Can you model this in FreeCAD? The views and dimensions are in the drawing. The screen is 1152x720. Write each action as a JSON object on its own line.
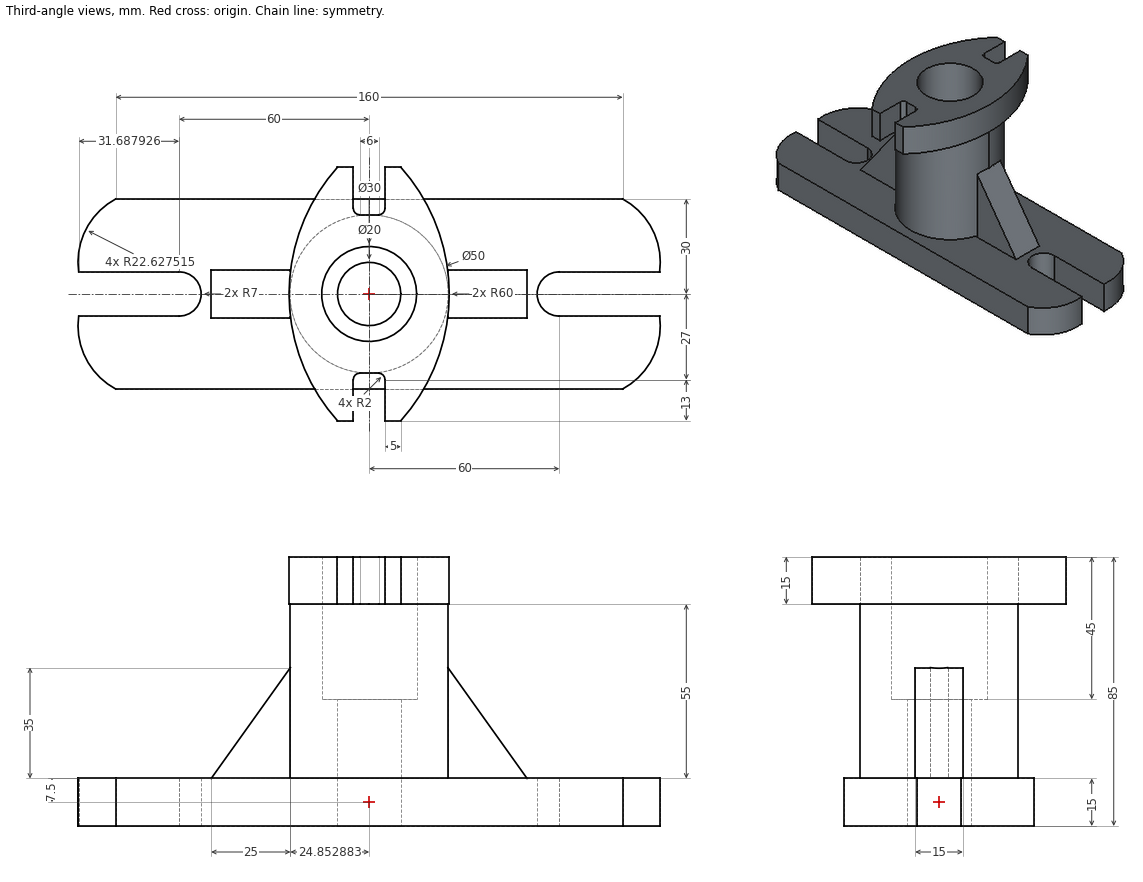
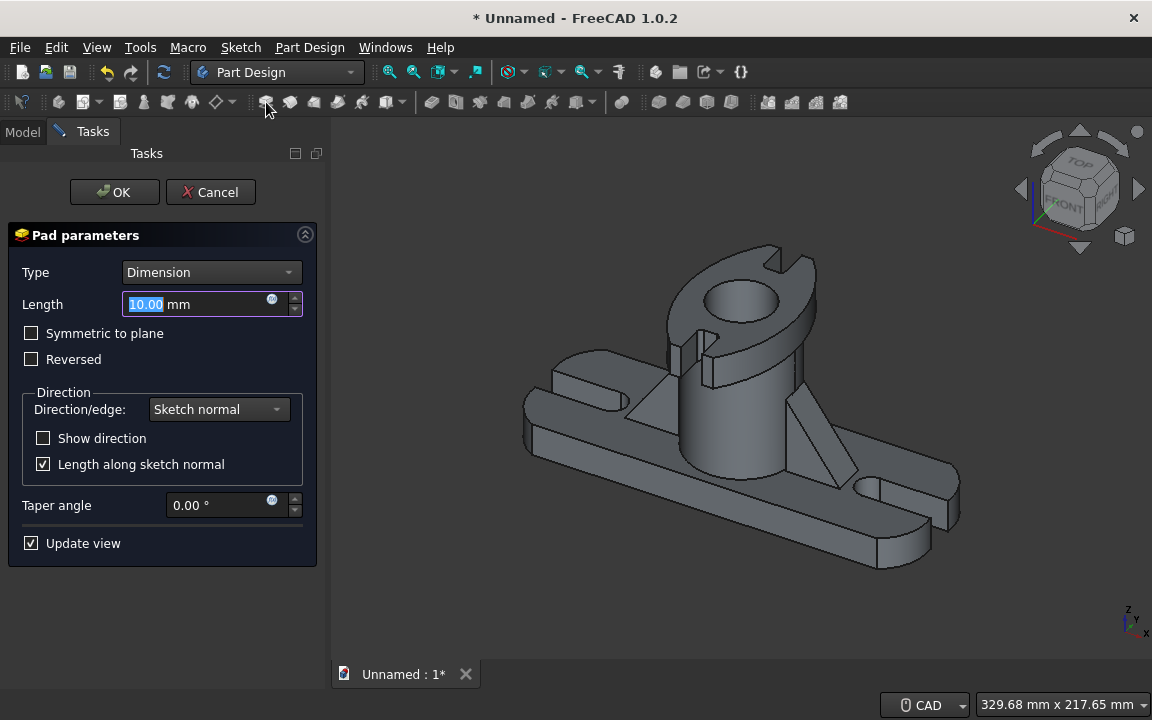
{"action": "type", "text": "85"}
{"action": "key", "text": "Tab"}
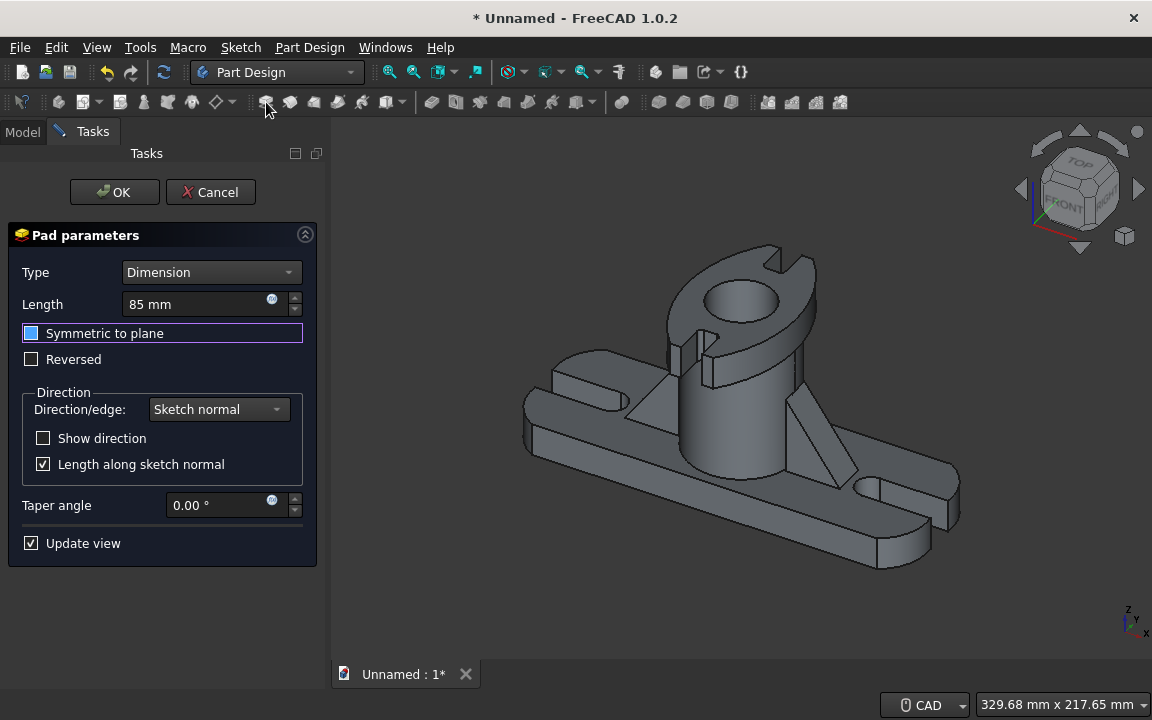
{"action": "left_click", "coordinate": [30, 359]}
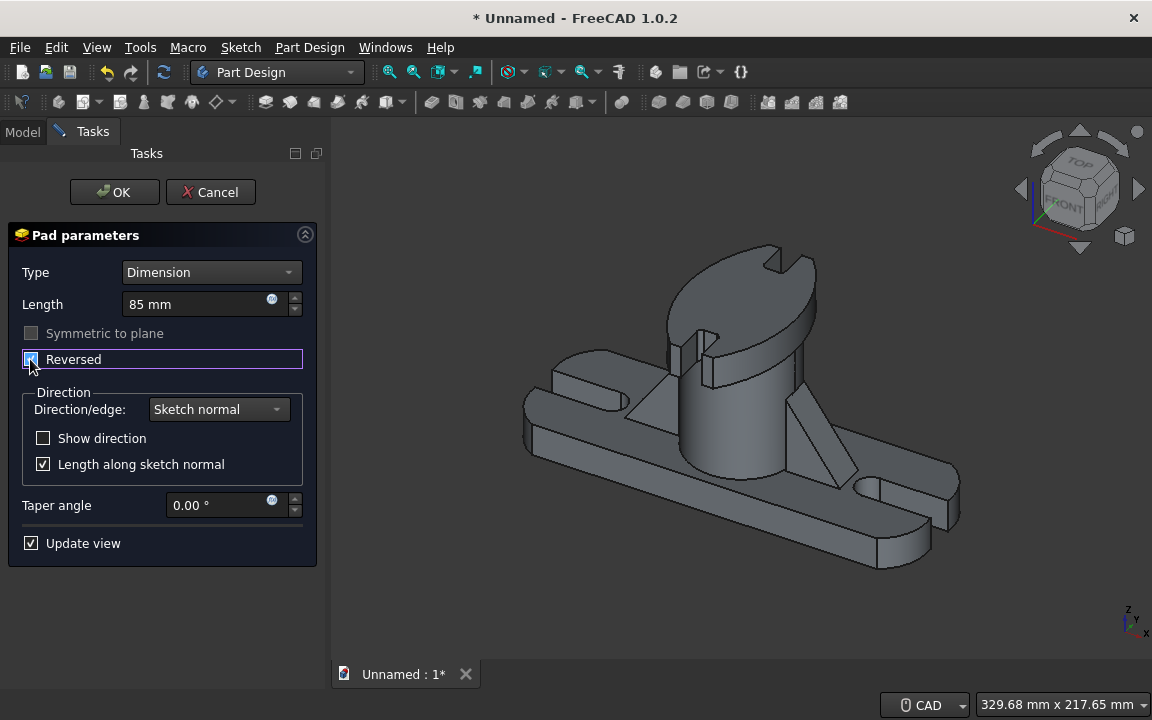
{"action": "left_click", "coordinate": [115, 192]}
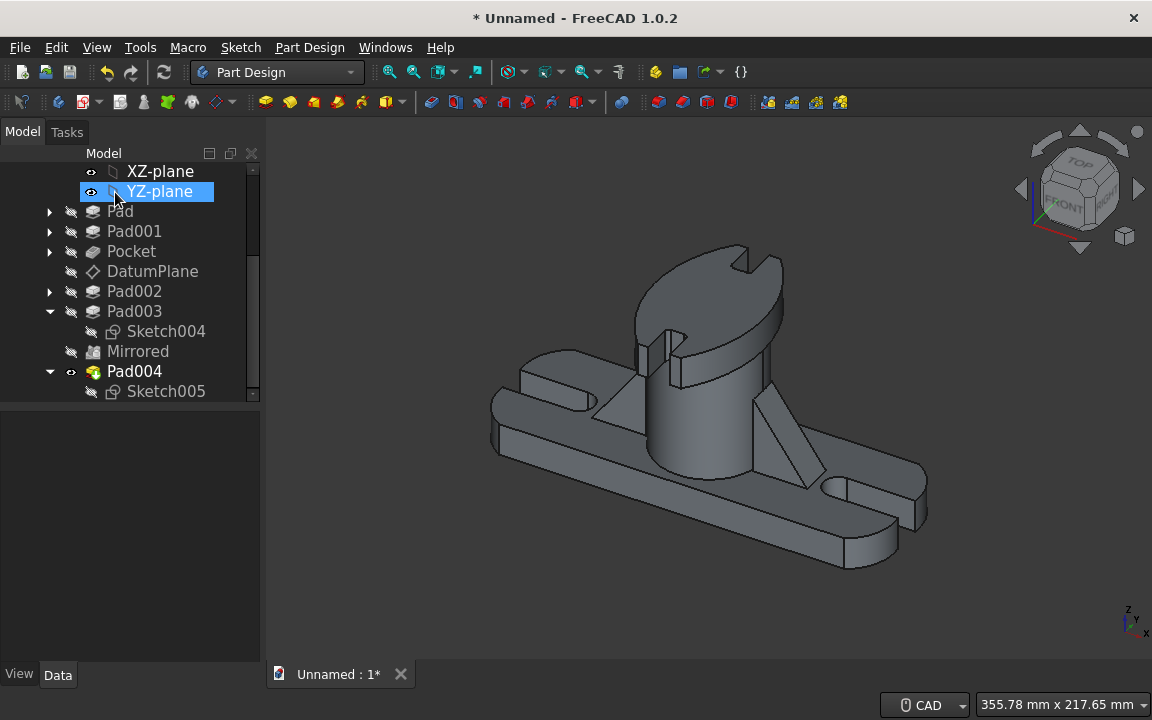
{"action": "left_click", "coordinate": [709, 300]}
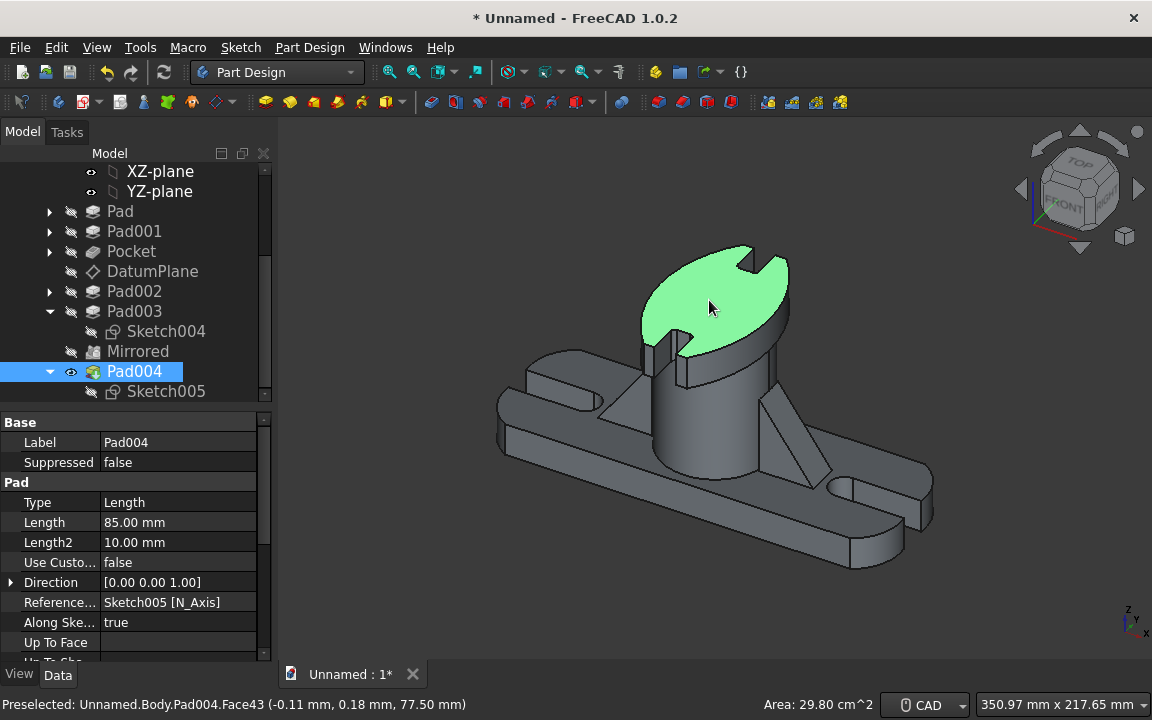
{"action": "left_click", "coordinate": [84, 102]}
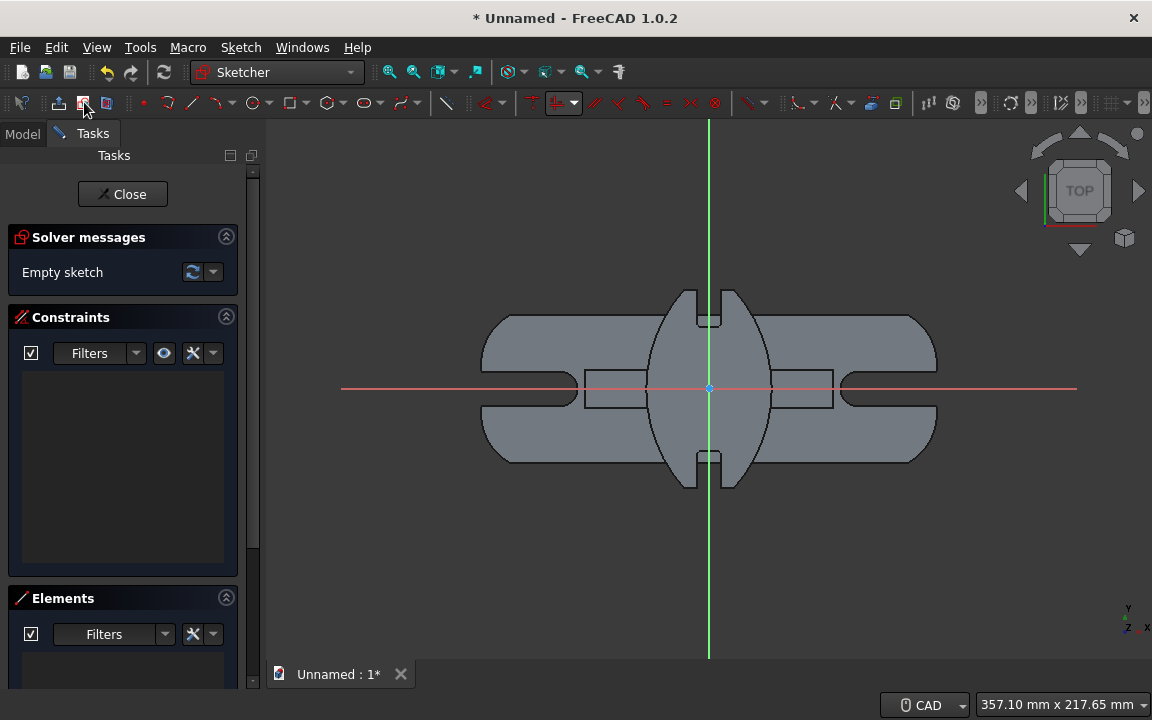
{"action": "scroll", "coordinate": [720, 389], "scroll_direction": "up", "scroll_amount": 10}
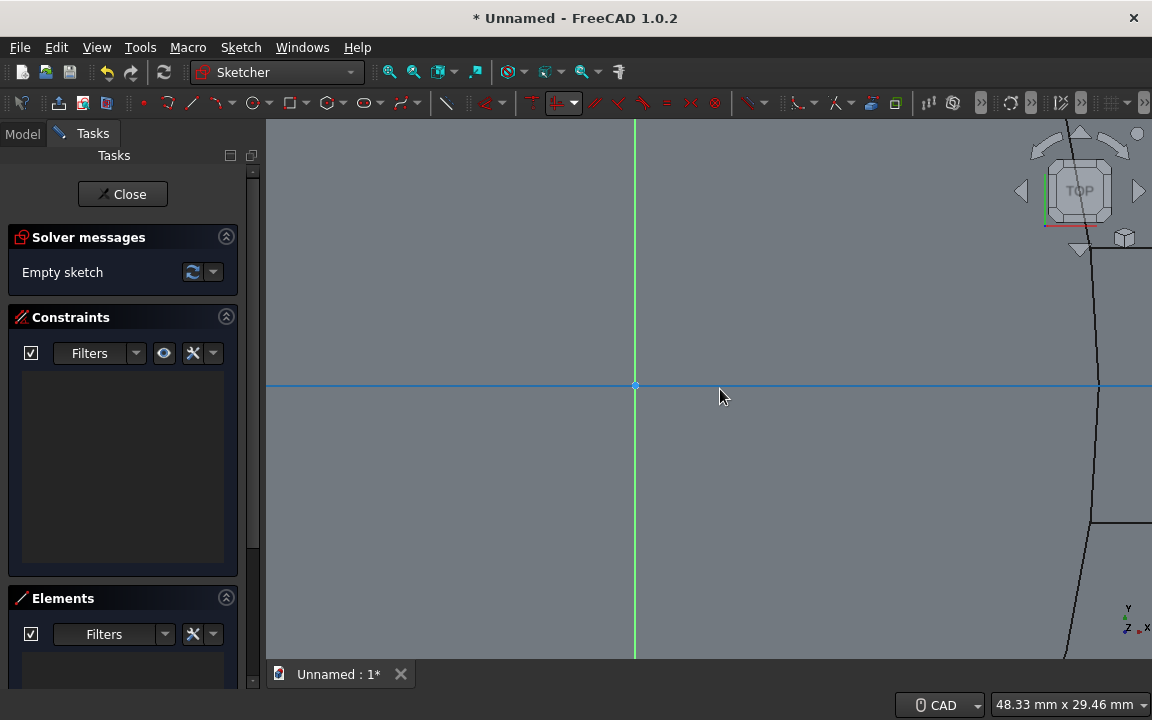
{"action": "key", "text": "g c"}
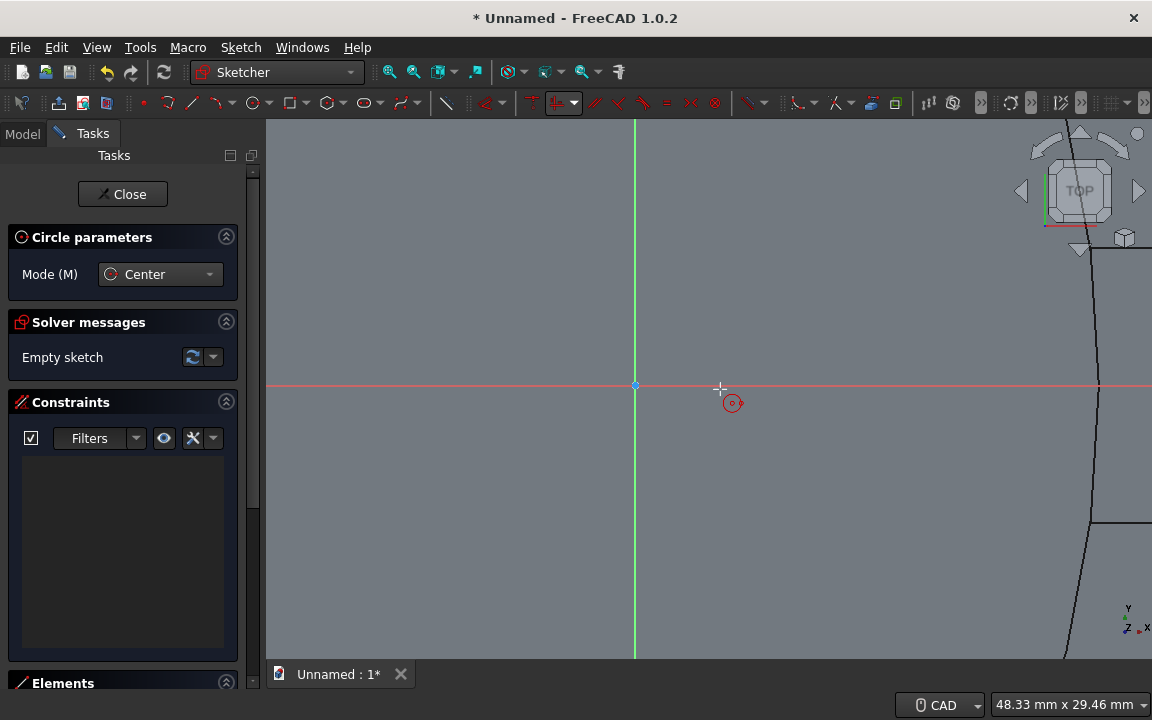
{"action": "left_click", "coordinate": [635, 386]}
{"action": "mouse_move", "coordinate": [765, 256]}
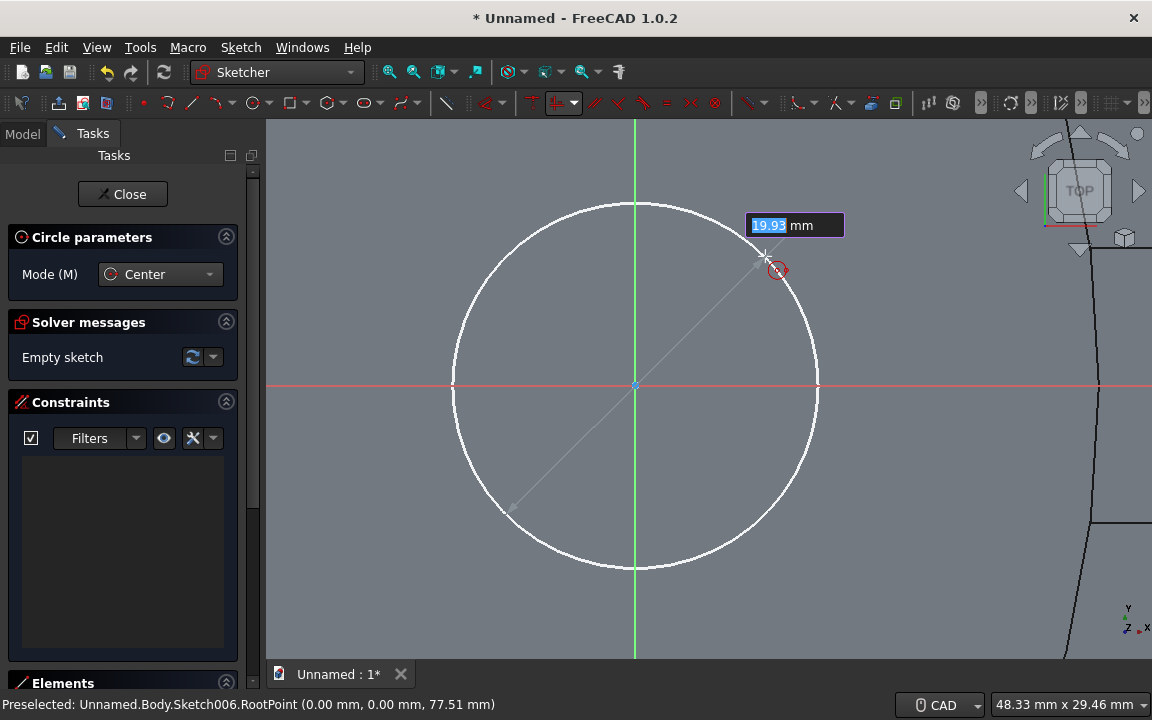
{"action": "type", "text": "20"}
{"action": "key", "text": "Return"}
{"action": "key", "text": "Escape"}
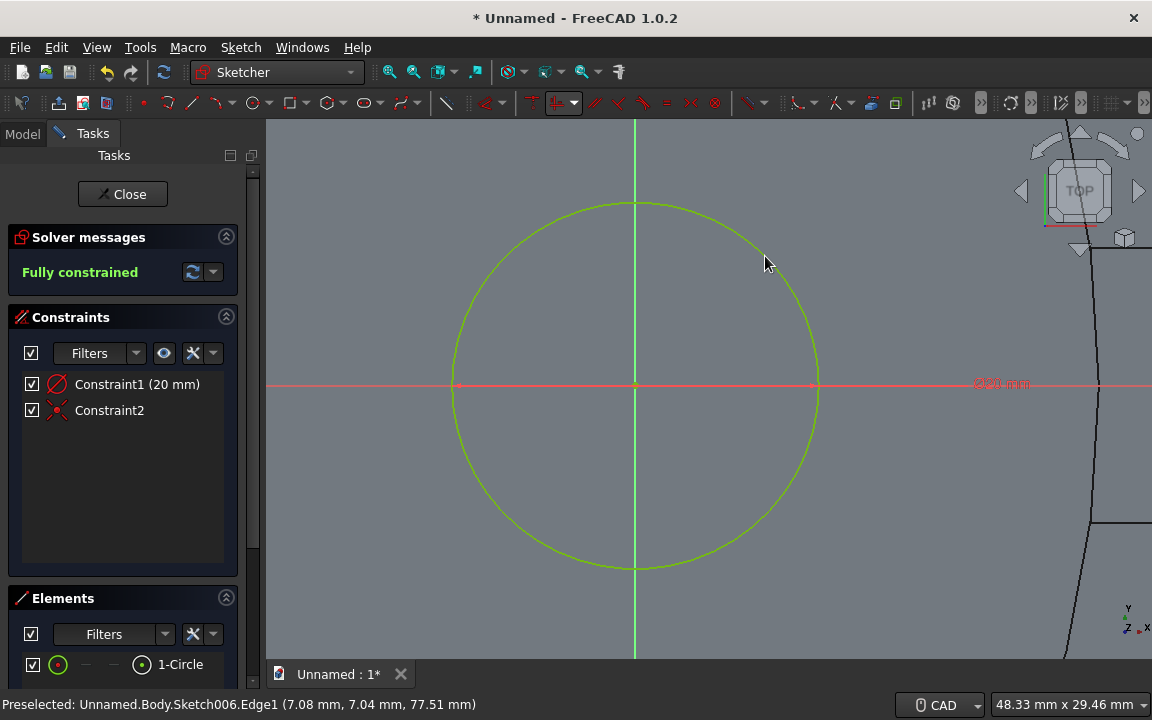
{"action": "left_click", "coordinate": [123, 194]}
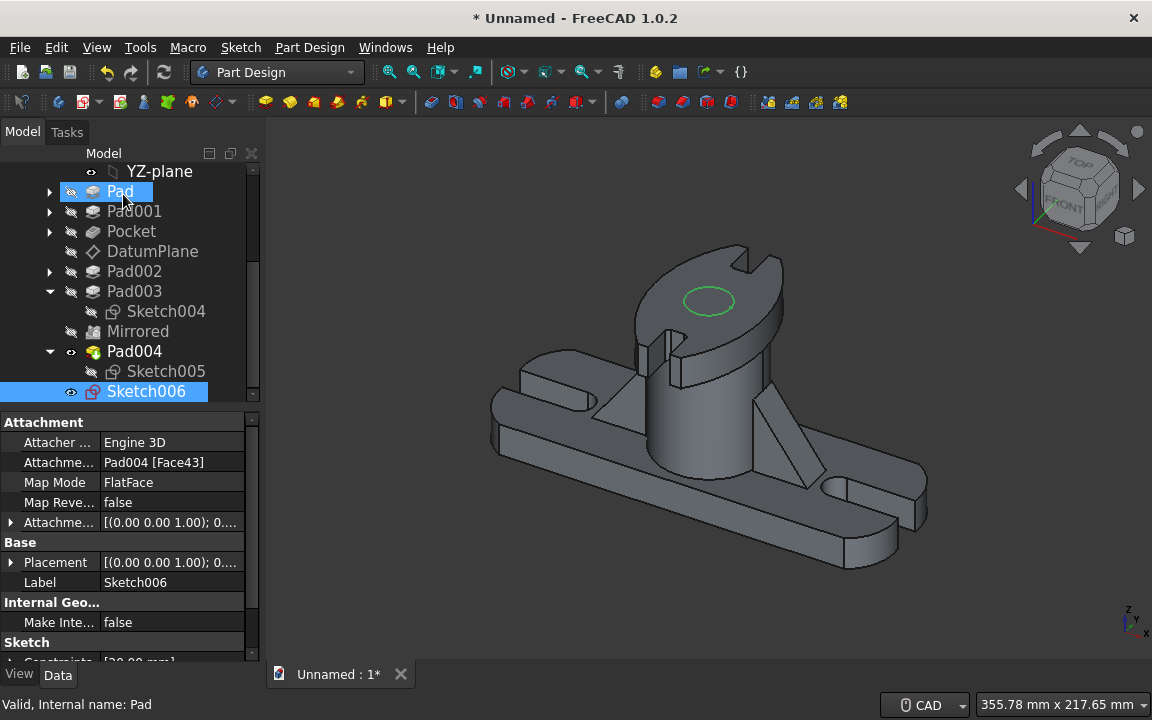
{"action": "left_click", "coordinate": [432, 102]}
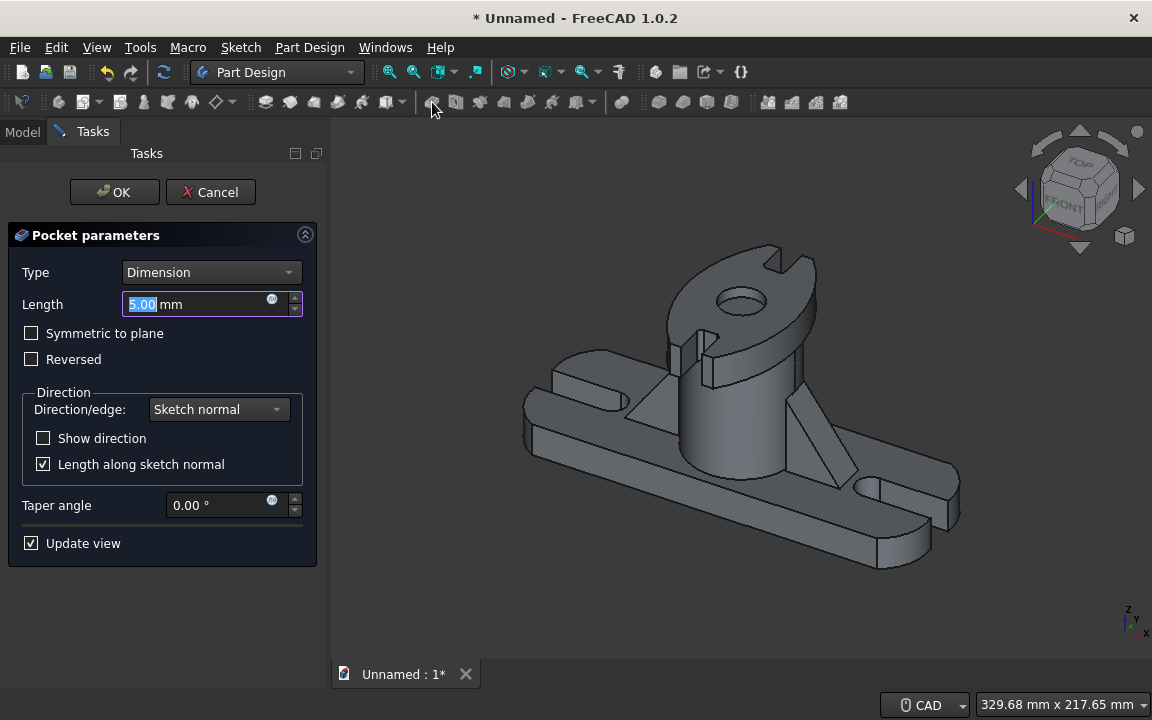
{"action": "left_click", "coordinate": [212, 272]}